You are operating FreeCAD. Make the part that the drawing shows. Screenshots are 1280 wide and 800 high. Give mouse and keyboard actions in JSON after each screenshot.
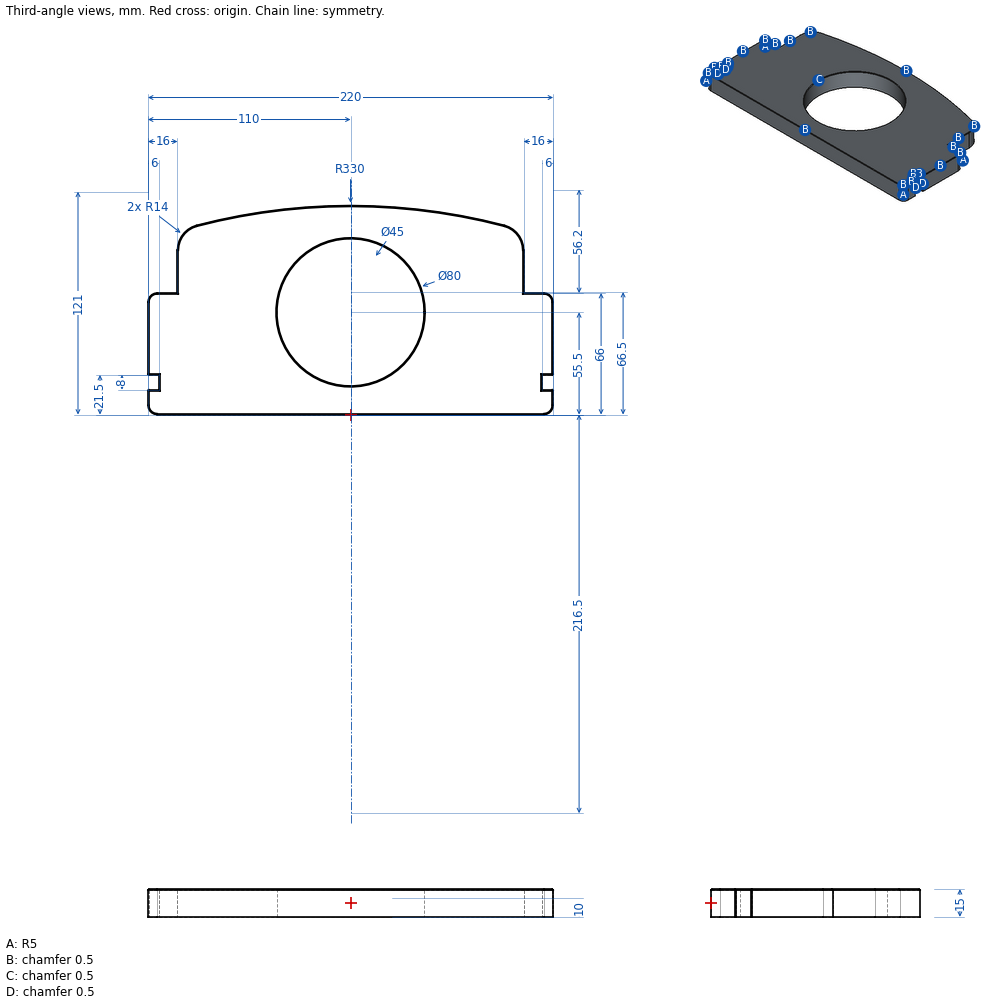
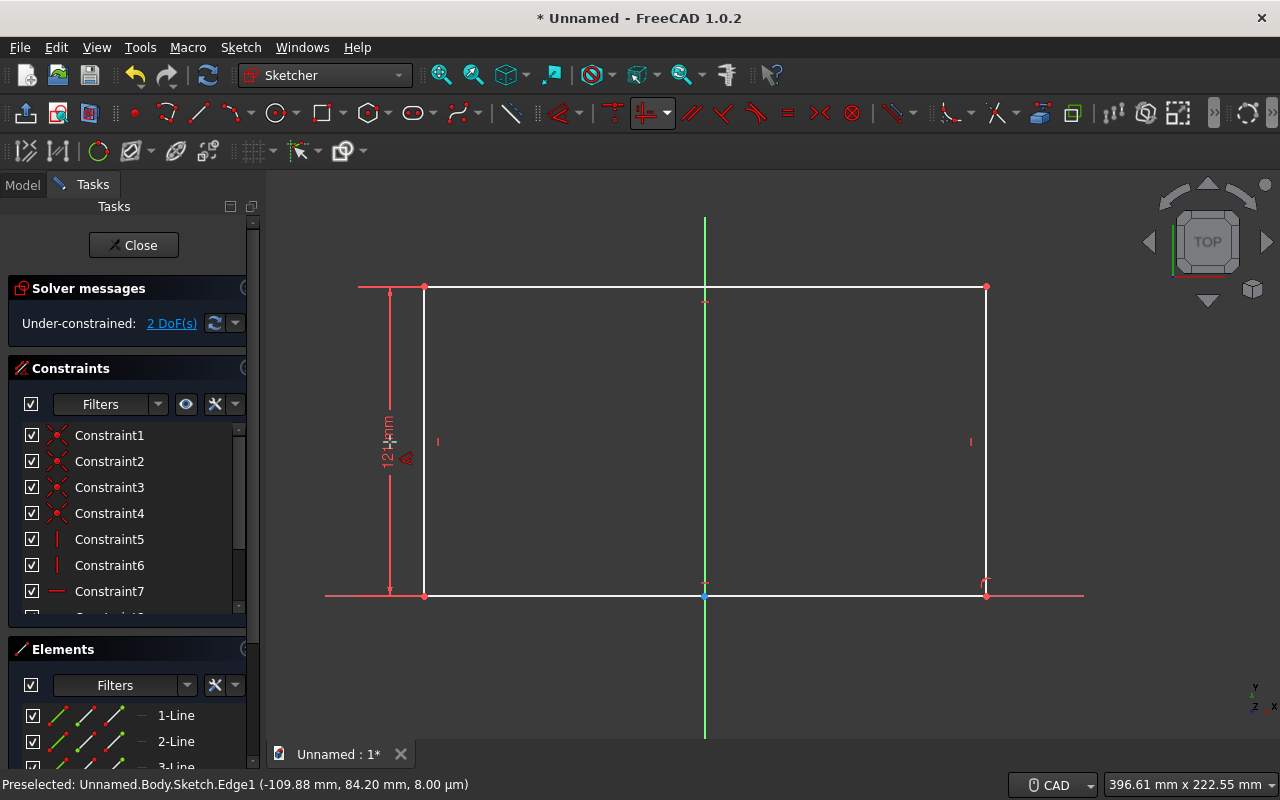
{"action": "left_click", "coordinate": [593, 596]}
{"action": "left_click", "coordinate": [576, 630]}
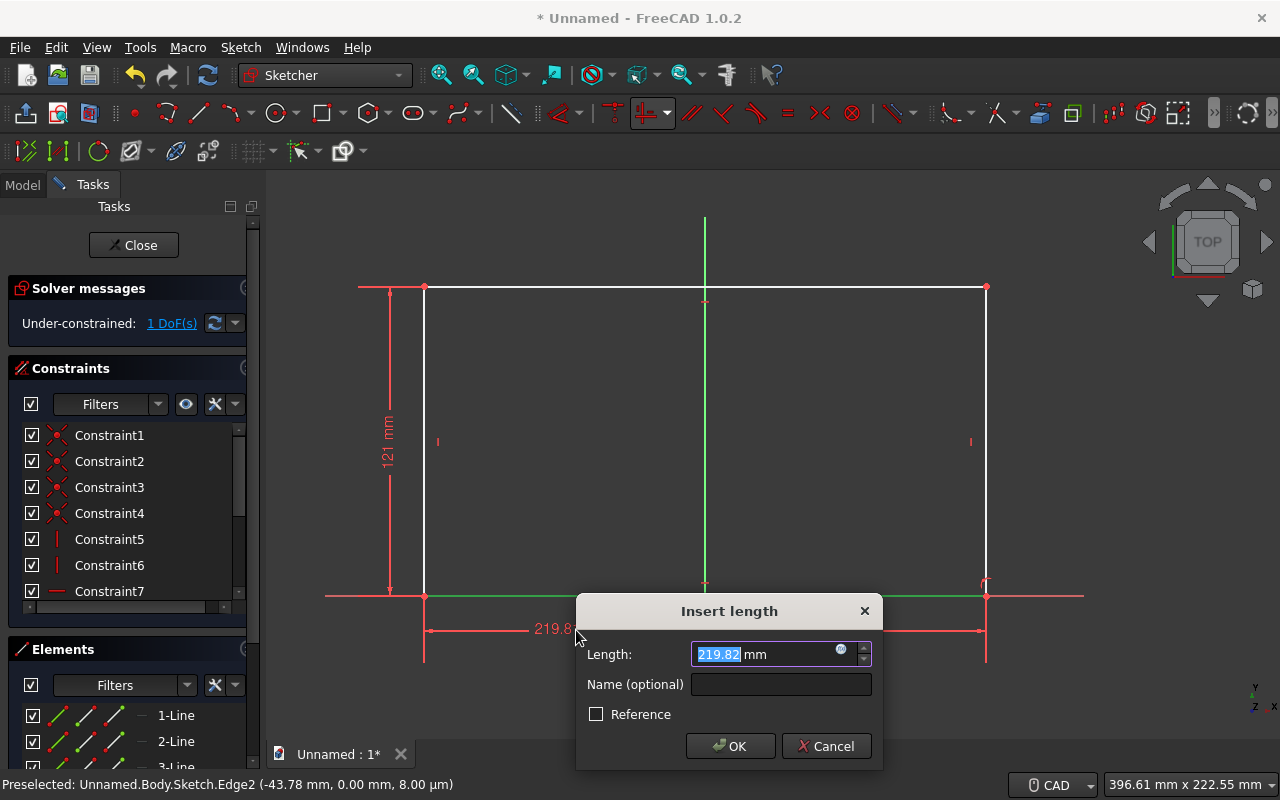
{"action": "type", "text": "220"}
{"action": "key", "text": "Return"}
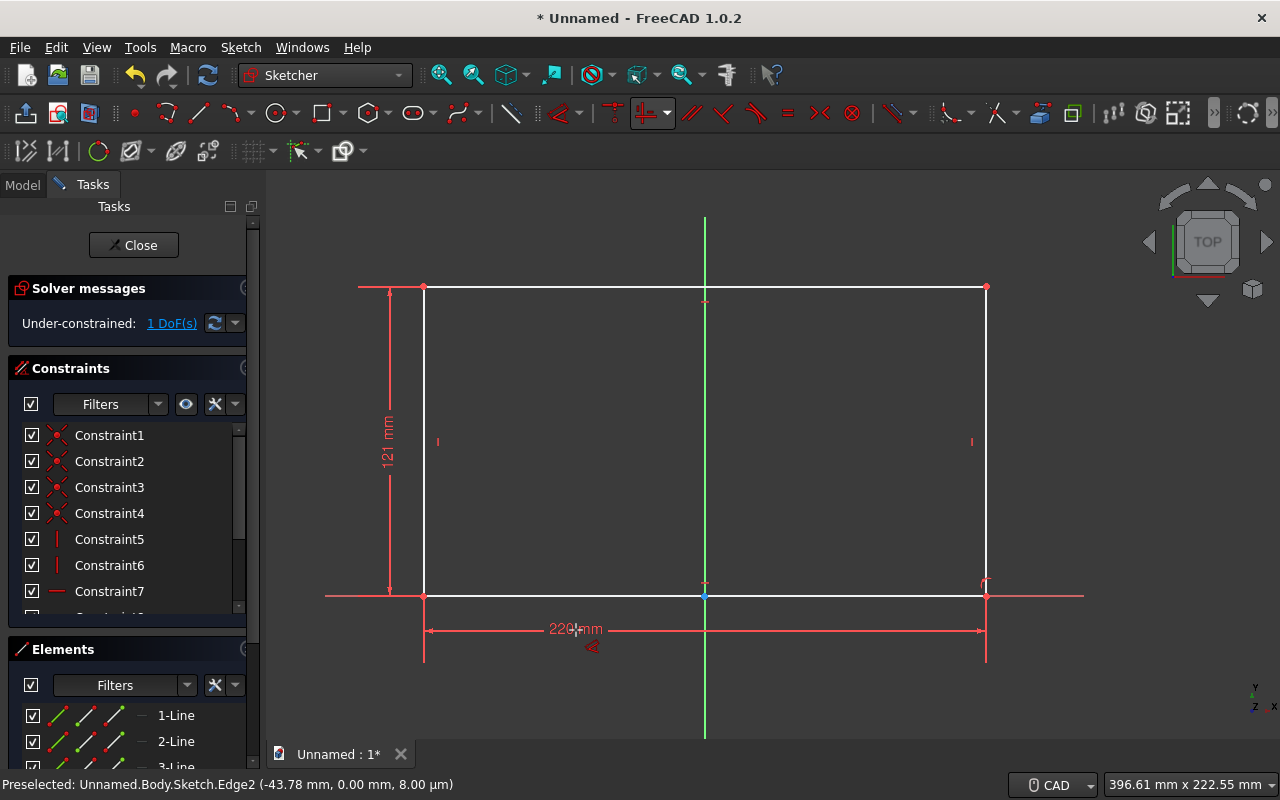
{"action": "left_click", "coordinate": [424, 287]}
{"action": "left_click", "coordinate": [500, 630]}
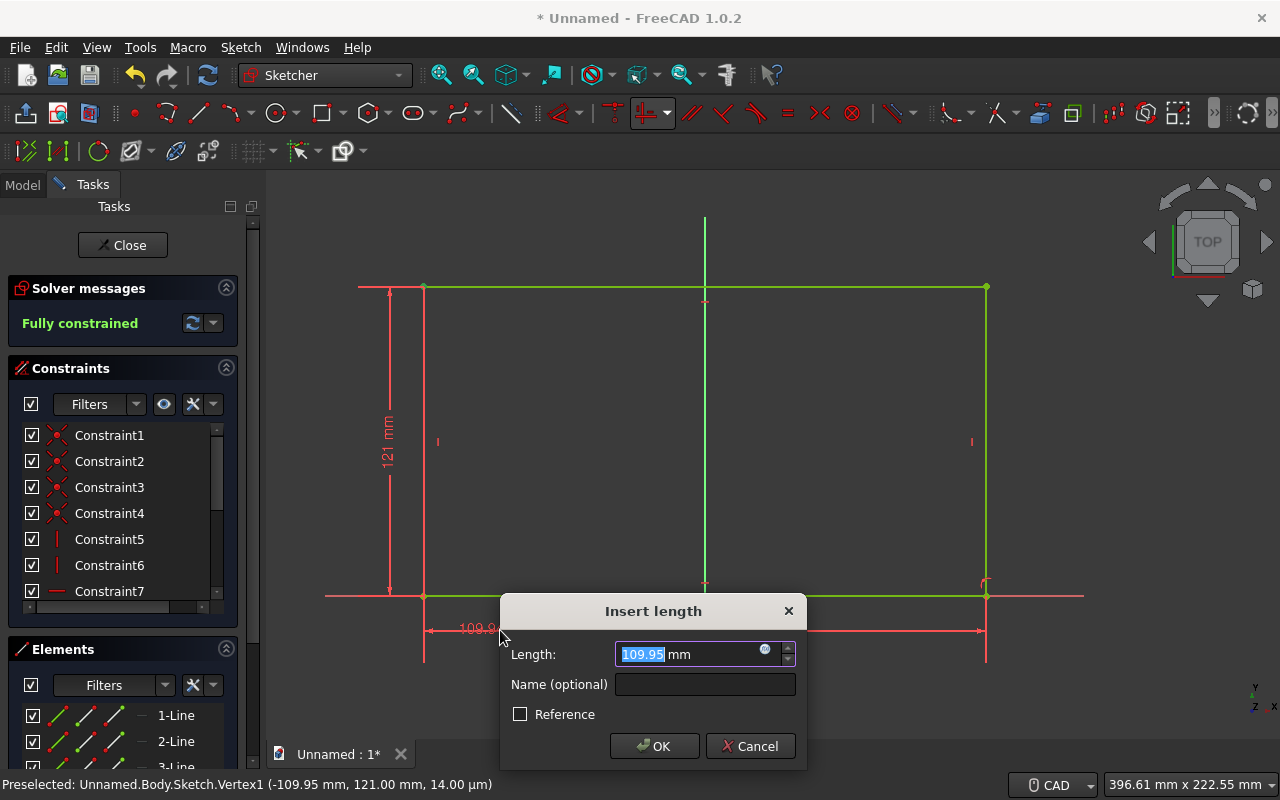
{"action": "type", "text": "110"}
{"action": "key", "text": "Return"}
{"action": "key", "text": "Escape"}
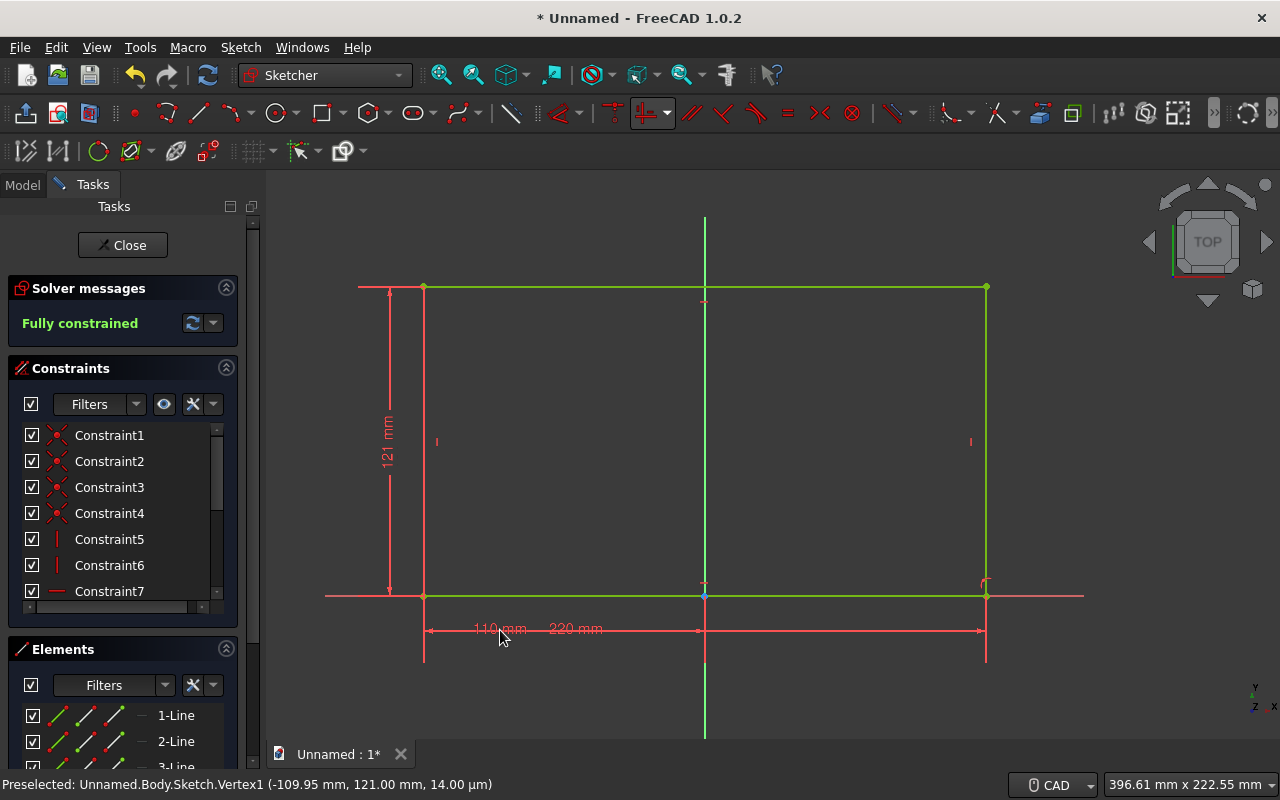
{"action": "left_click", "coordinate": [123, 245]}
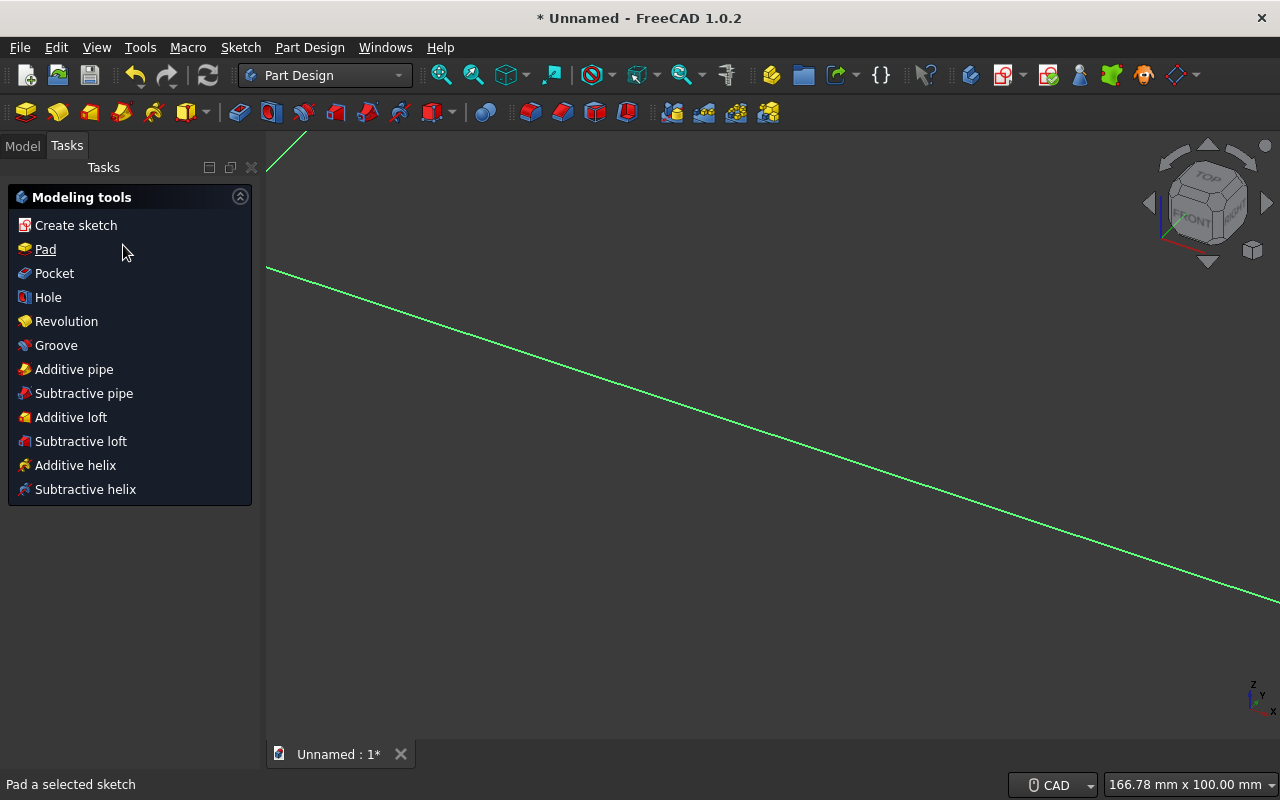
{"action": "left_click", "coordinate": [26, 112]}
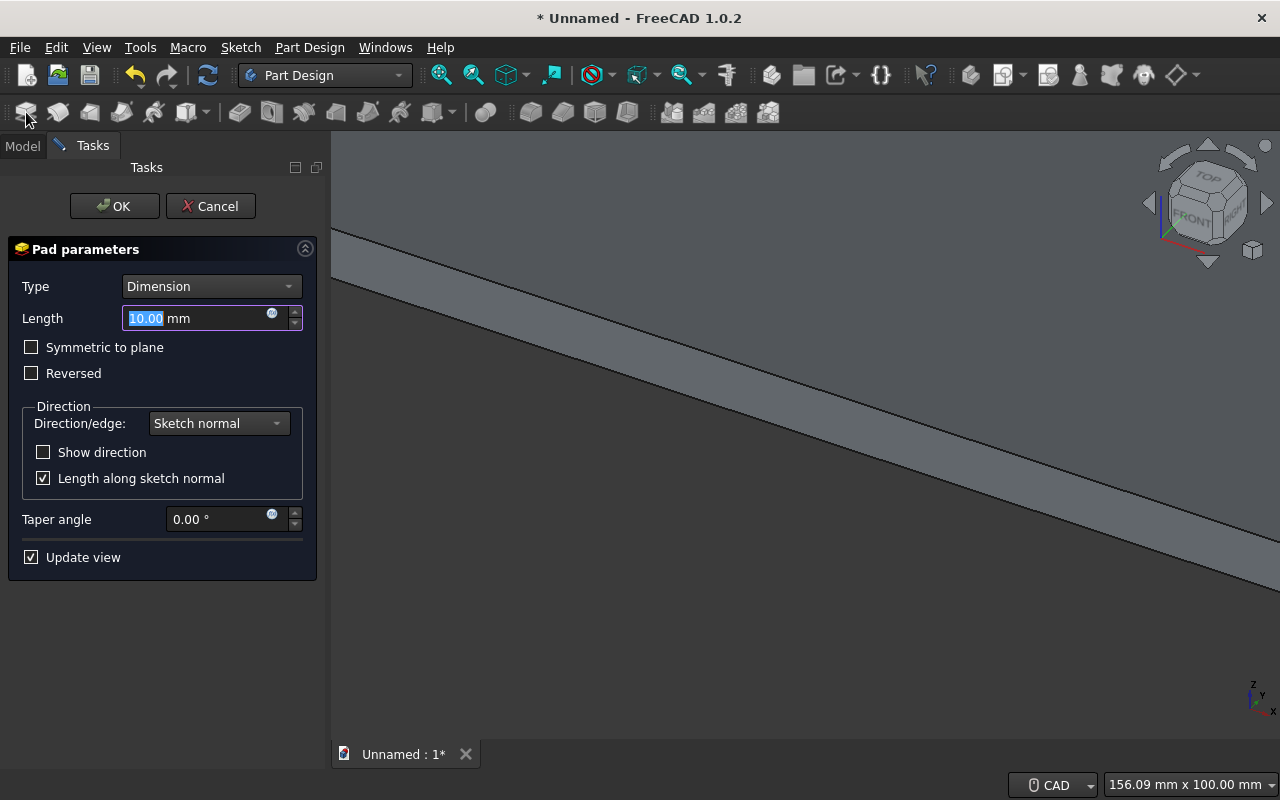
{"action": "type", "text": "15"}
{"action": "key", "text": "Tab"}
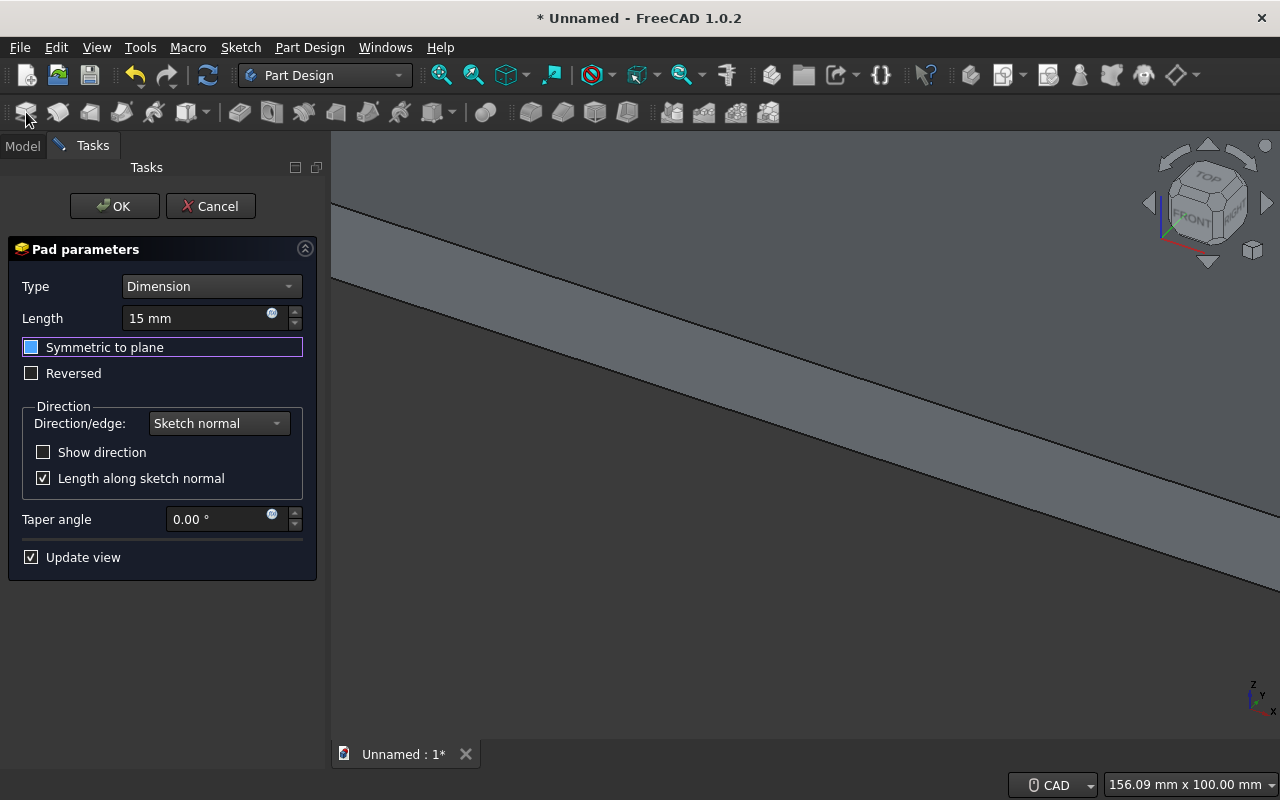
{"action": "left_click", "coordinate": [30, 347]}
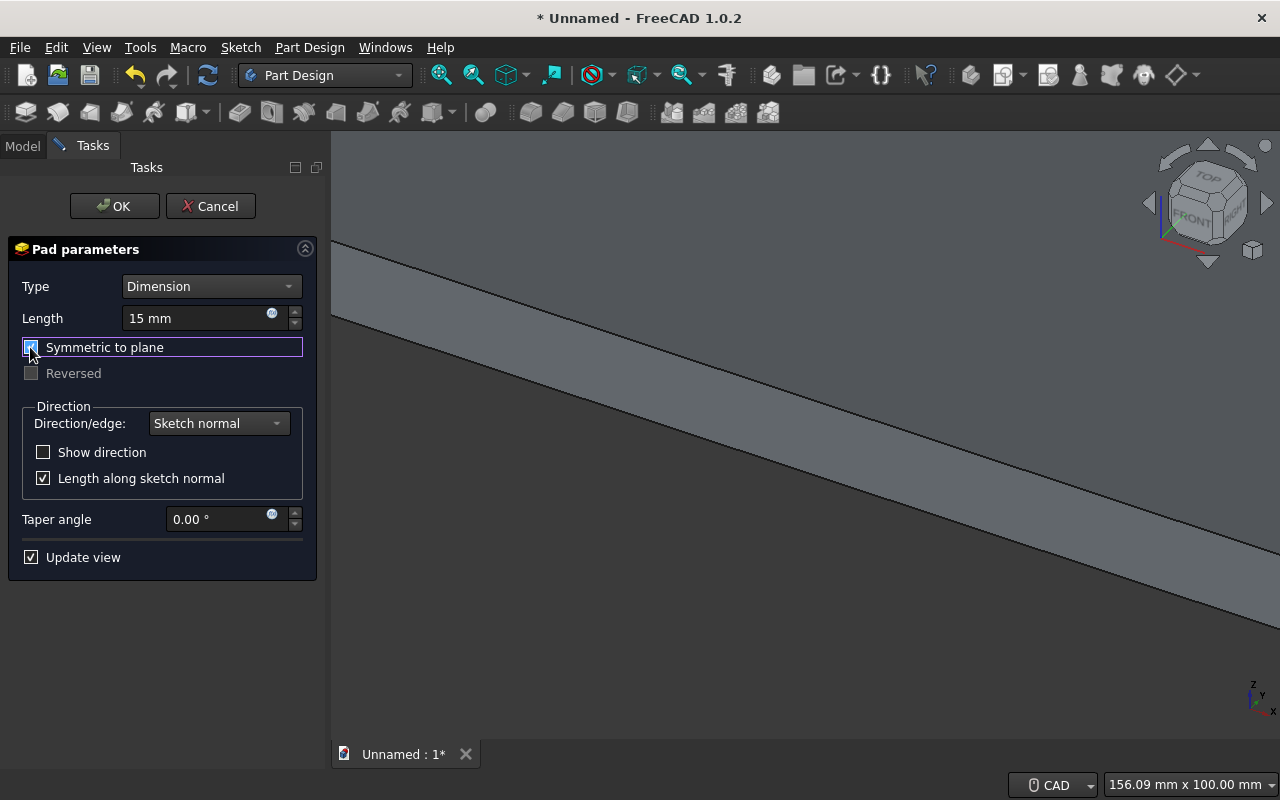
{"action": "left_click", "coordinate": [115, 206]}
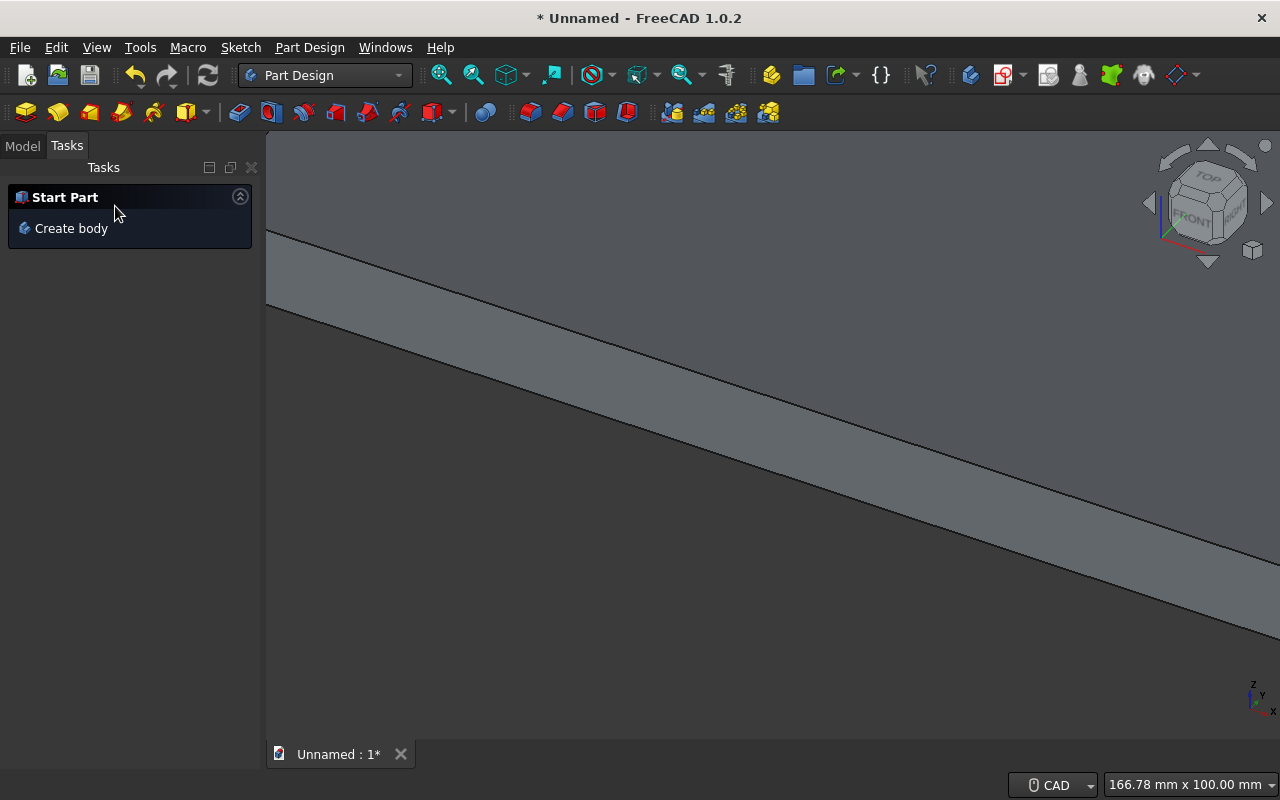
{"action": "left_click", "coordinate": [442, 76]}